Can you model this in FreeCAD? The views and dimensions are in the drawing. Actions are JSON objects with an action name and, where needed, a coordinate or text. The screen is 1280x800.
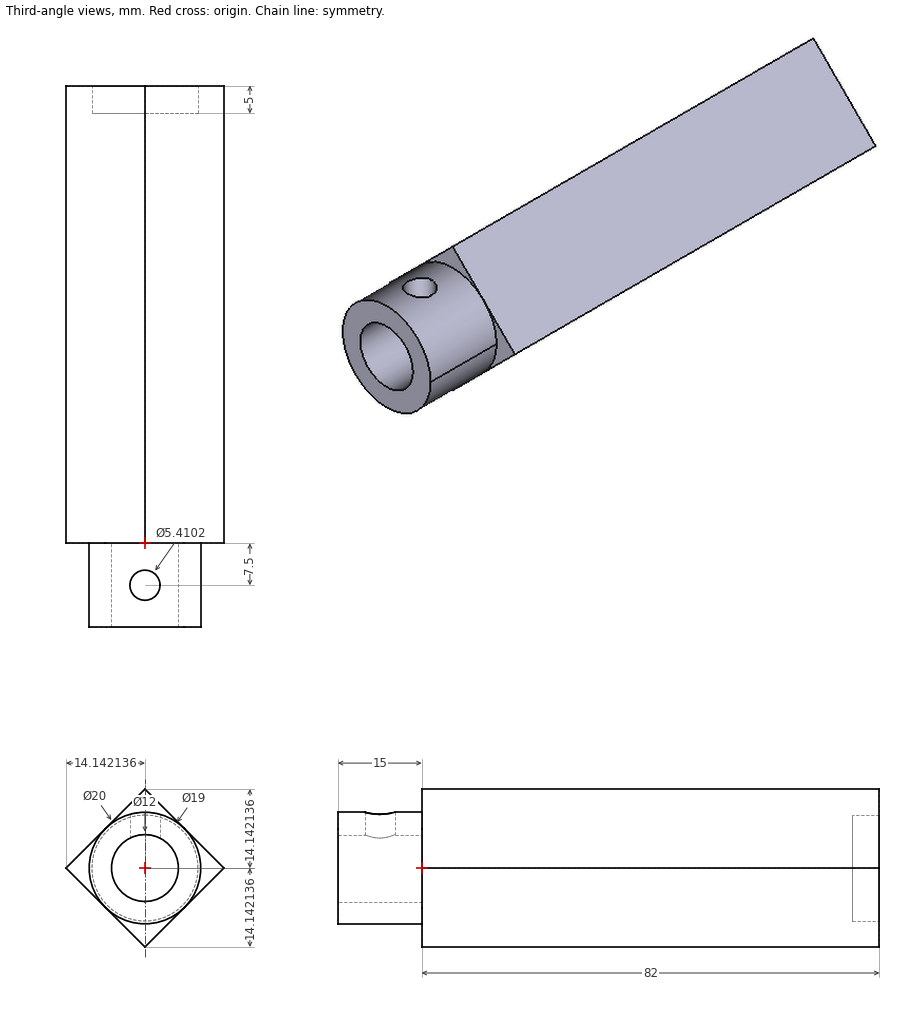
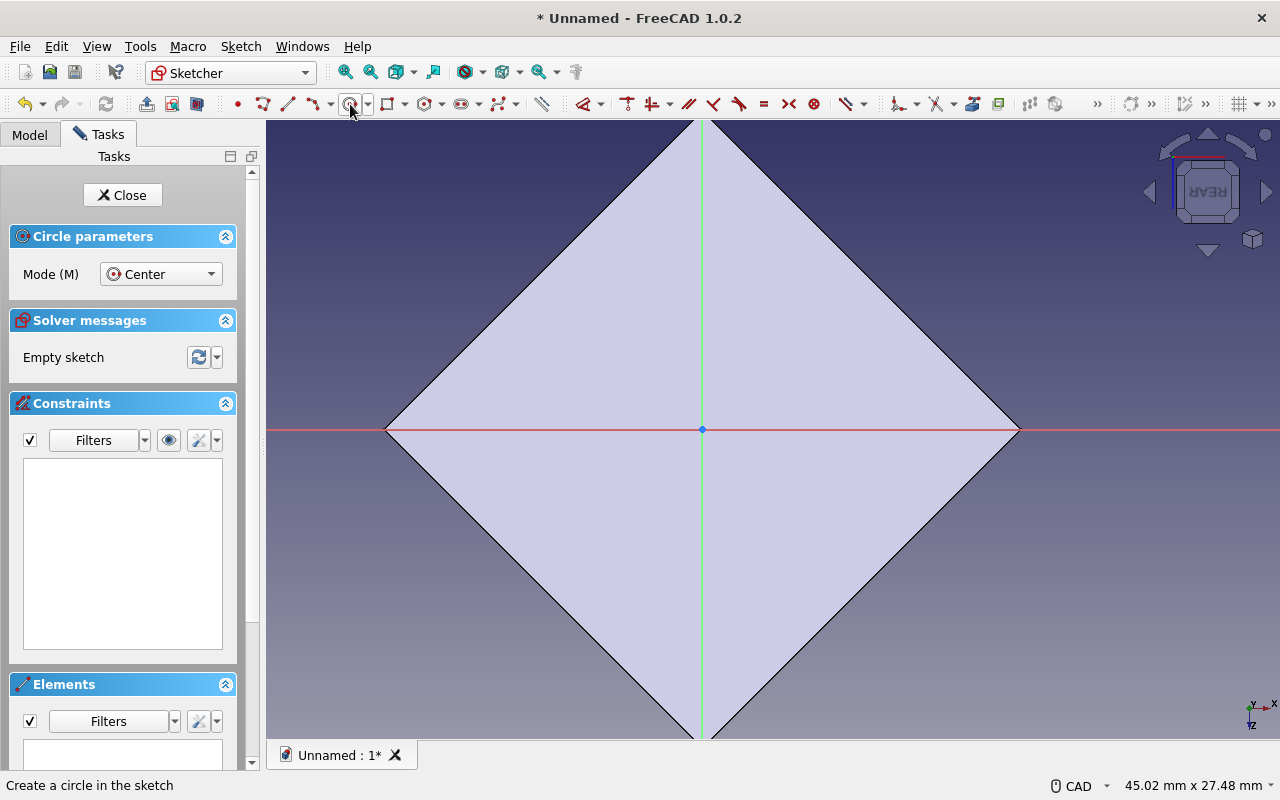
{"action": "left_click", "coordinate": [702, 429]}
{"action": "mouse_move", "coordinate": [853, 278]}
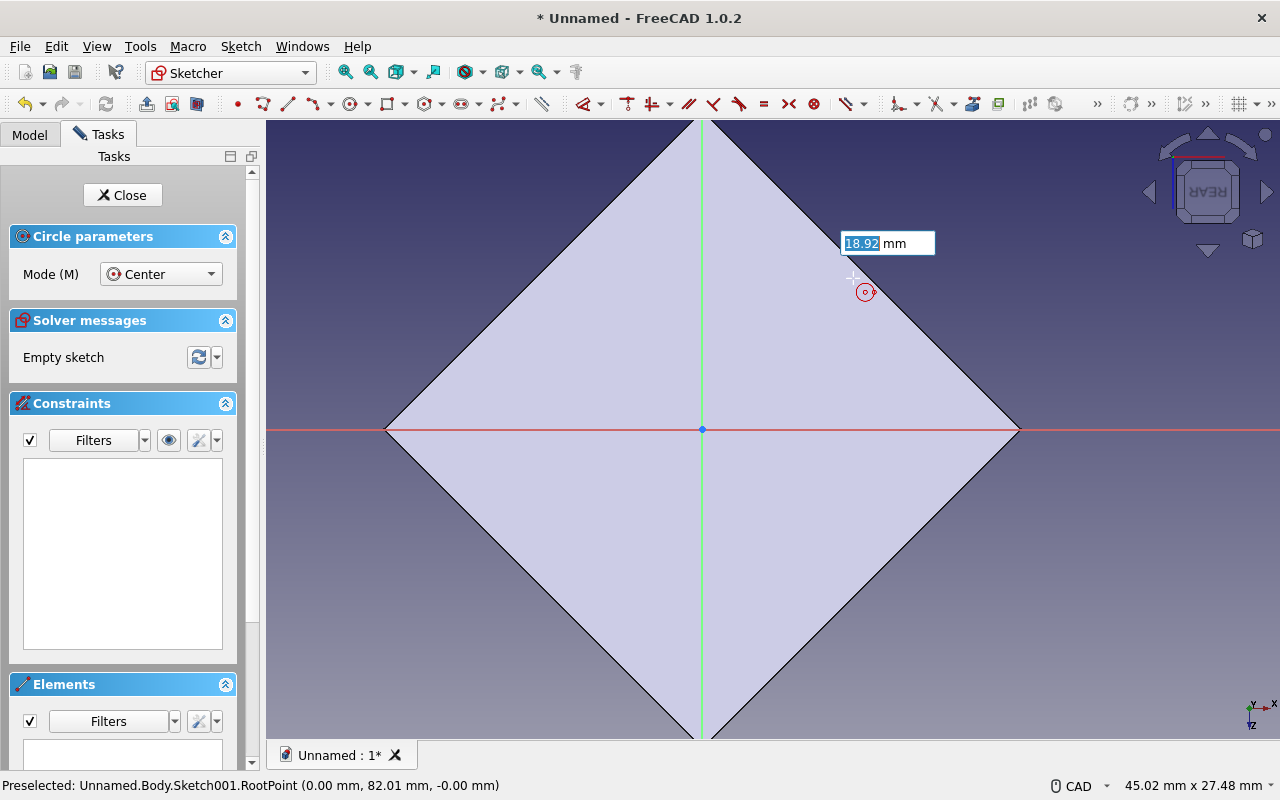
{"action": "type", "text": "19"}
{"action": "key", "text": "Return"}
{"action": "key", "text": "Escape"}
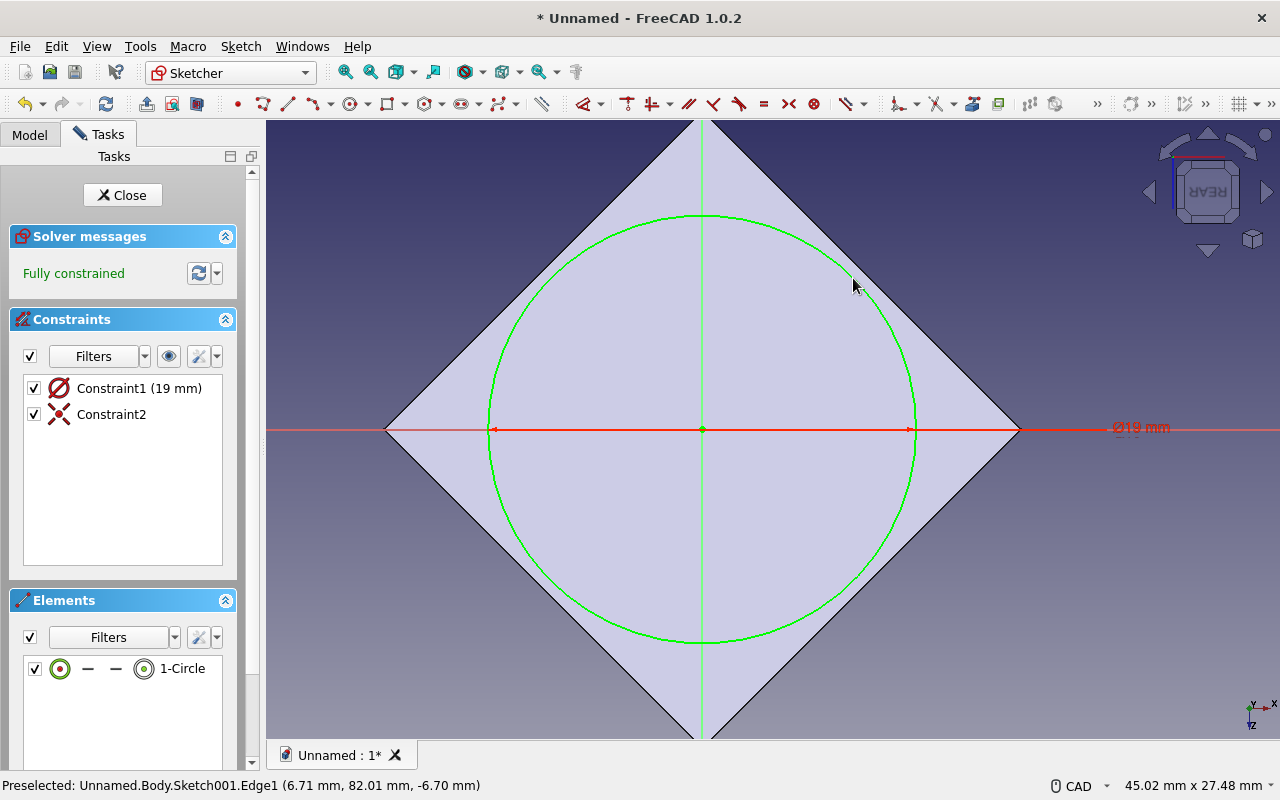
{"action": "left_click", "coordinate": [123, 195]}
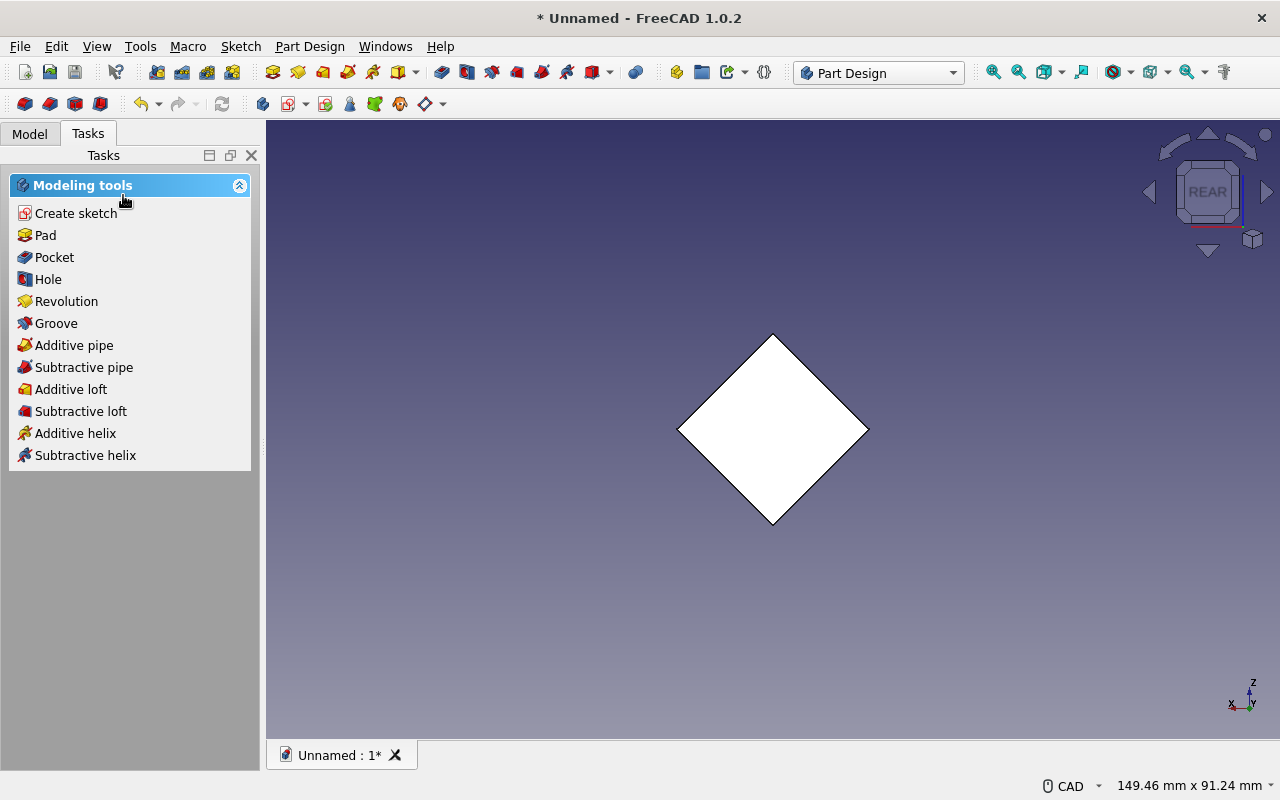
{"action": "left_click", "coordinate": [442, 72]}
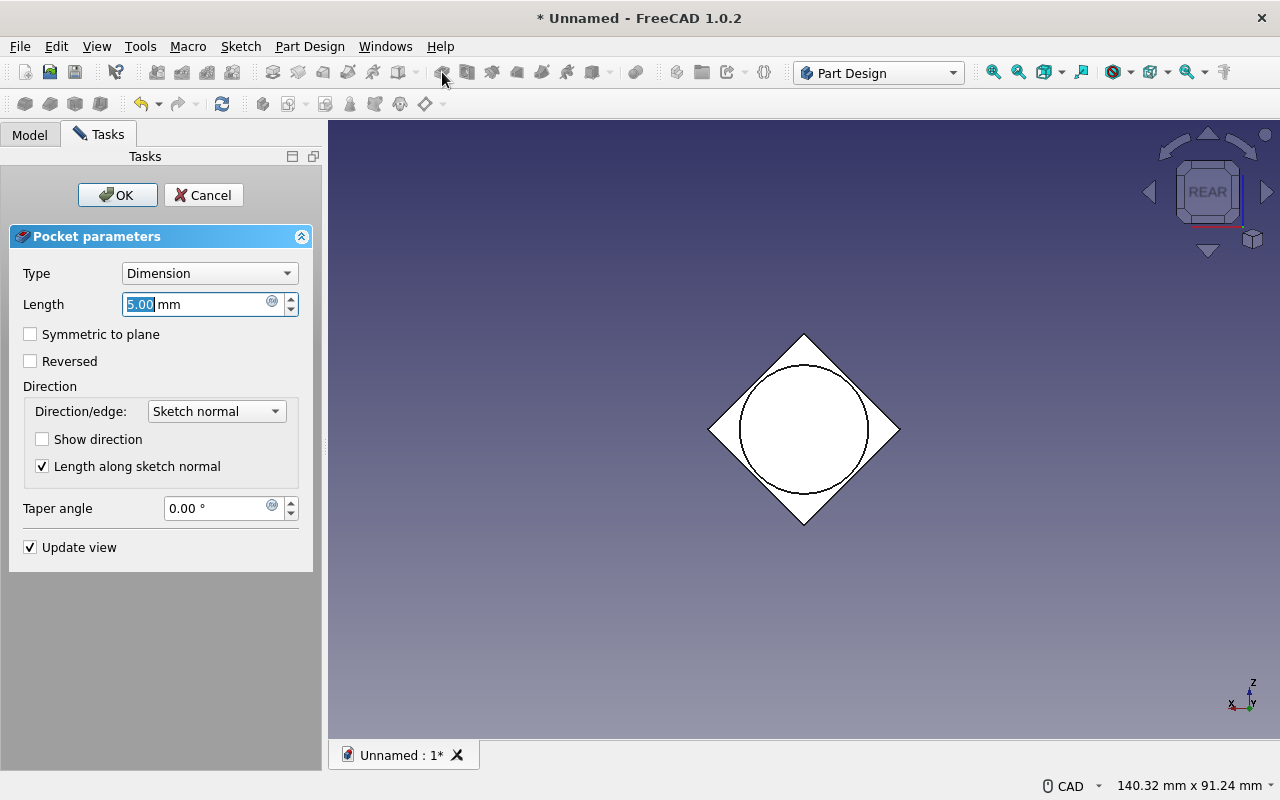
{"action": "type", "text": "5"}
{"action": "key", "text": "Tab"}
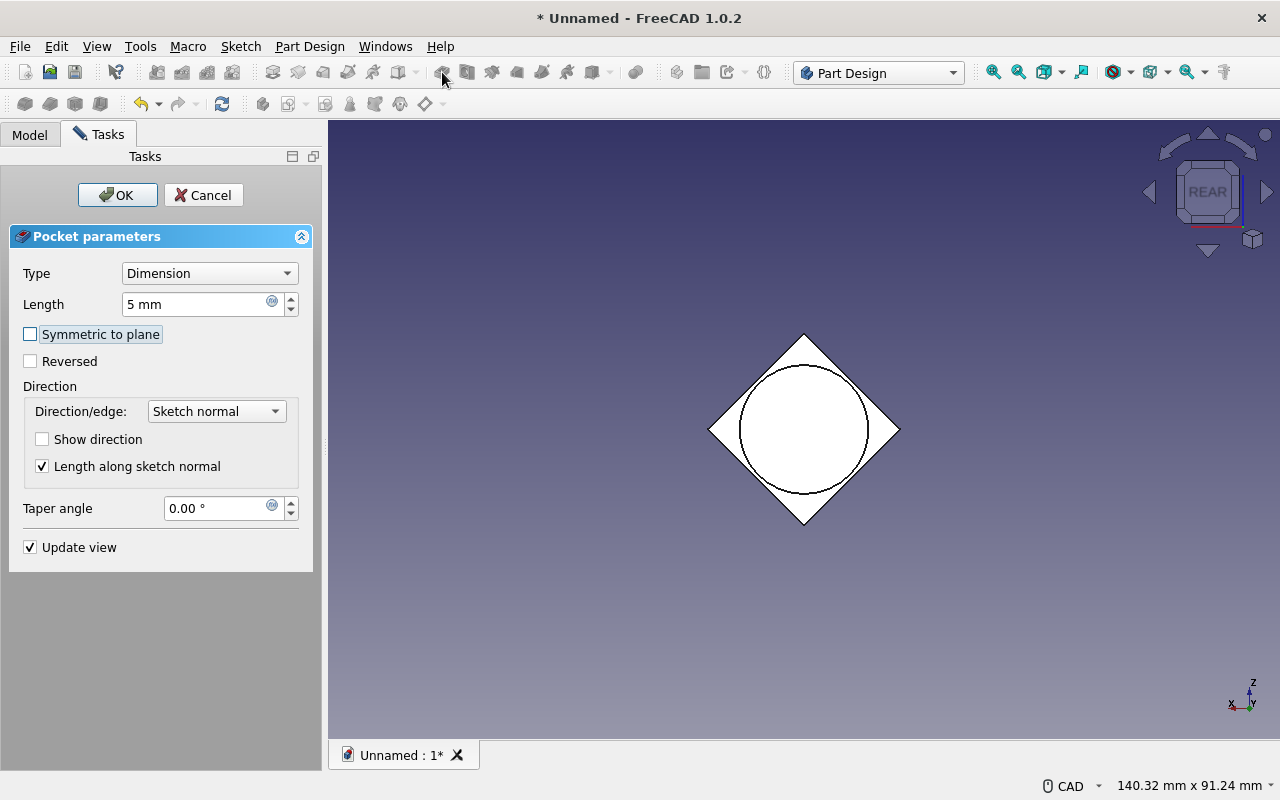
{"action": "left_click", "coordinate": [118, 195]}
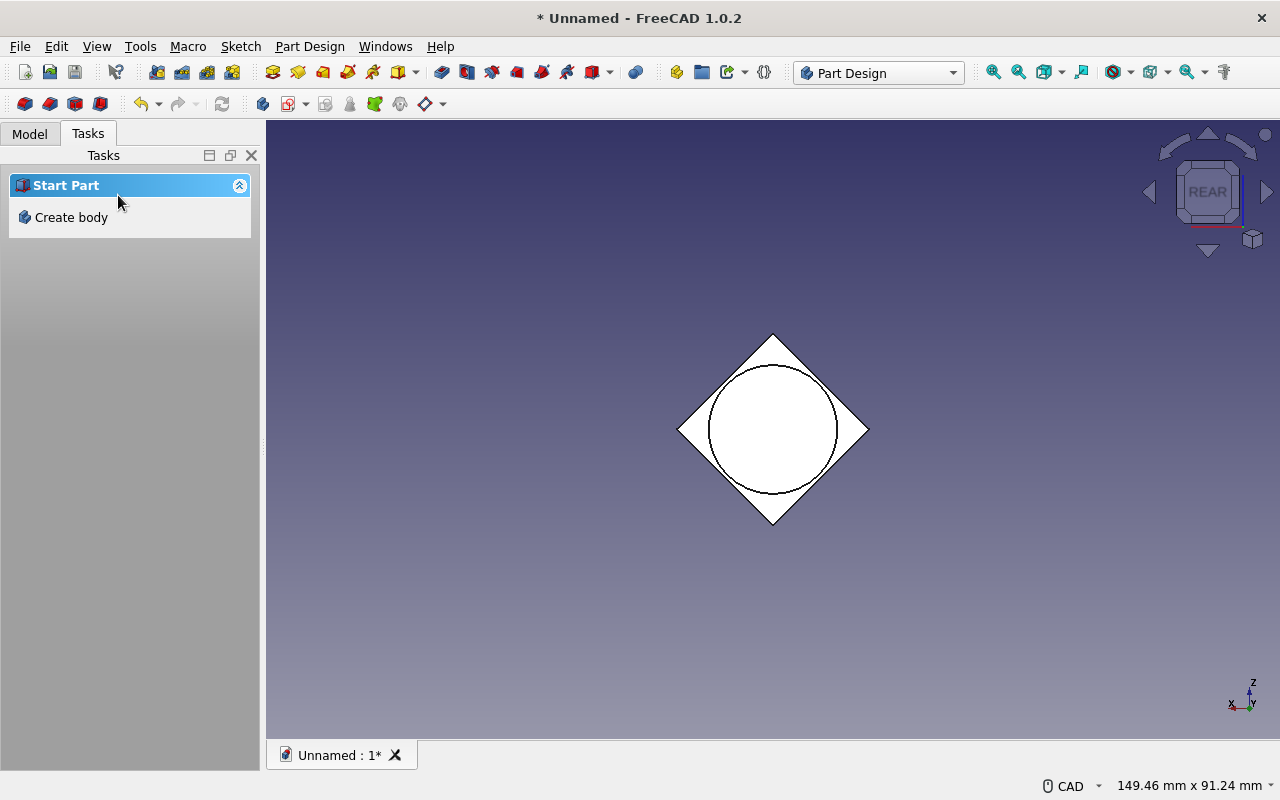
{"action": "key", "text": "v f"}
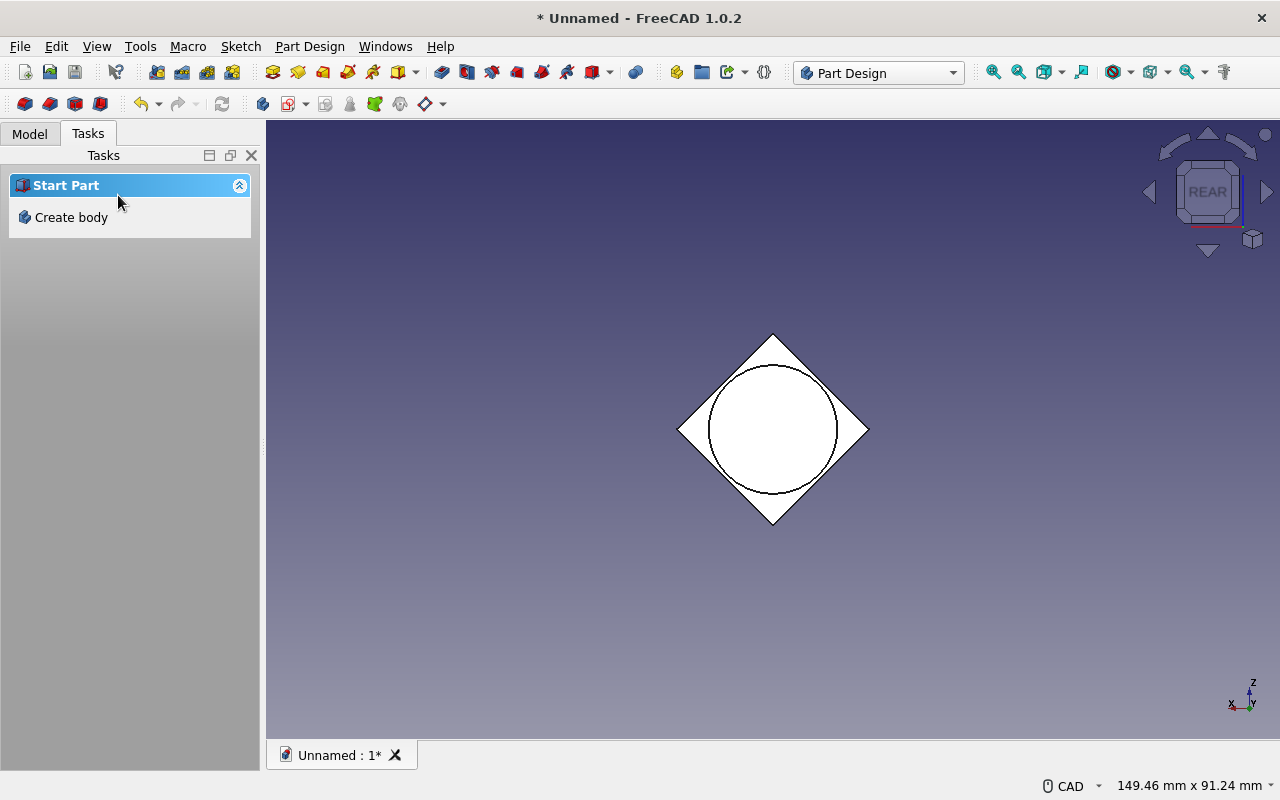
{"action": "key", "text": "0"}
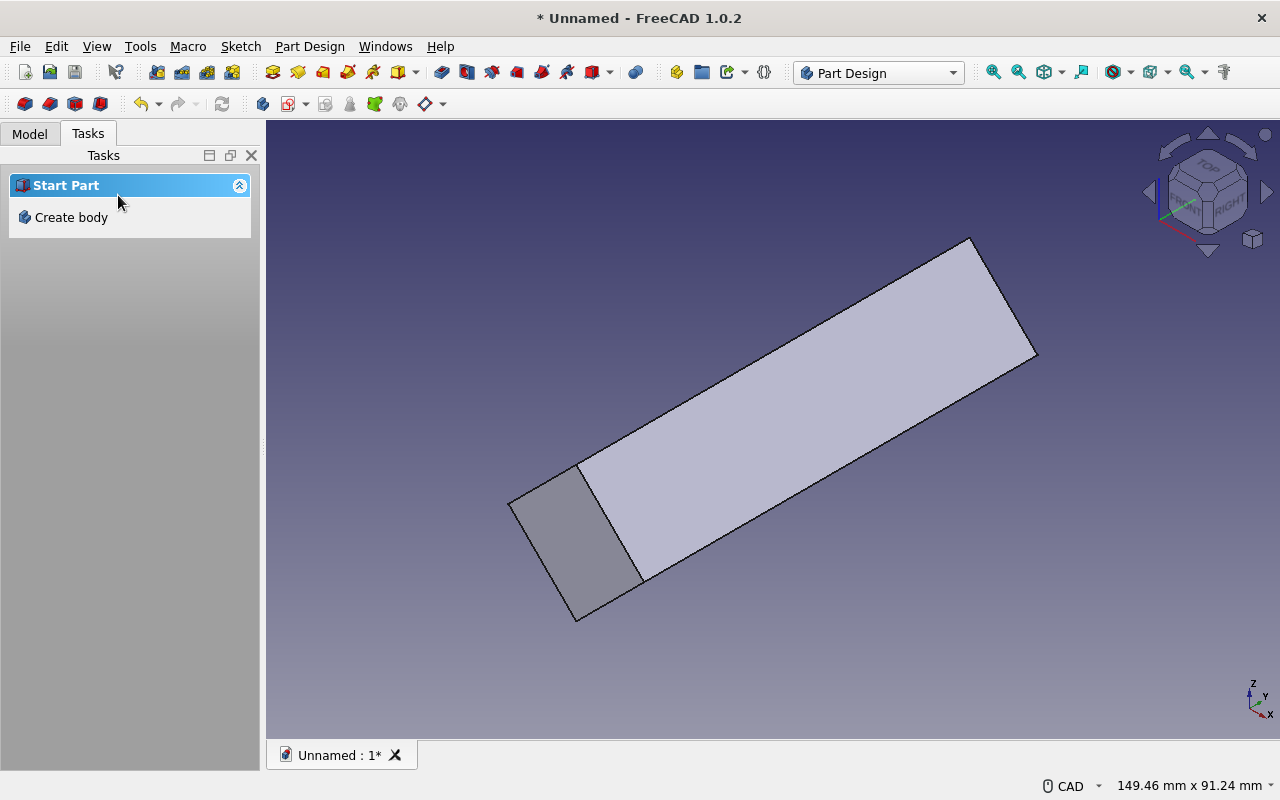
{"action": "left_click", "coordinate": [576, 542]}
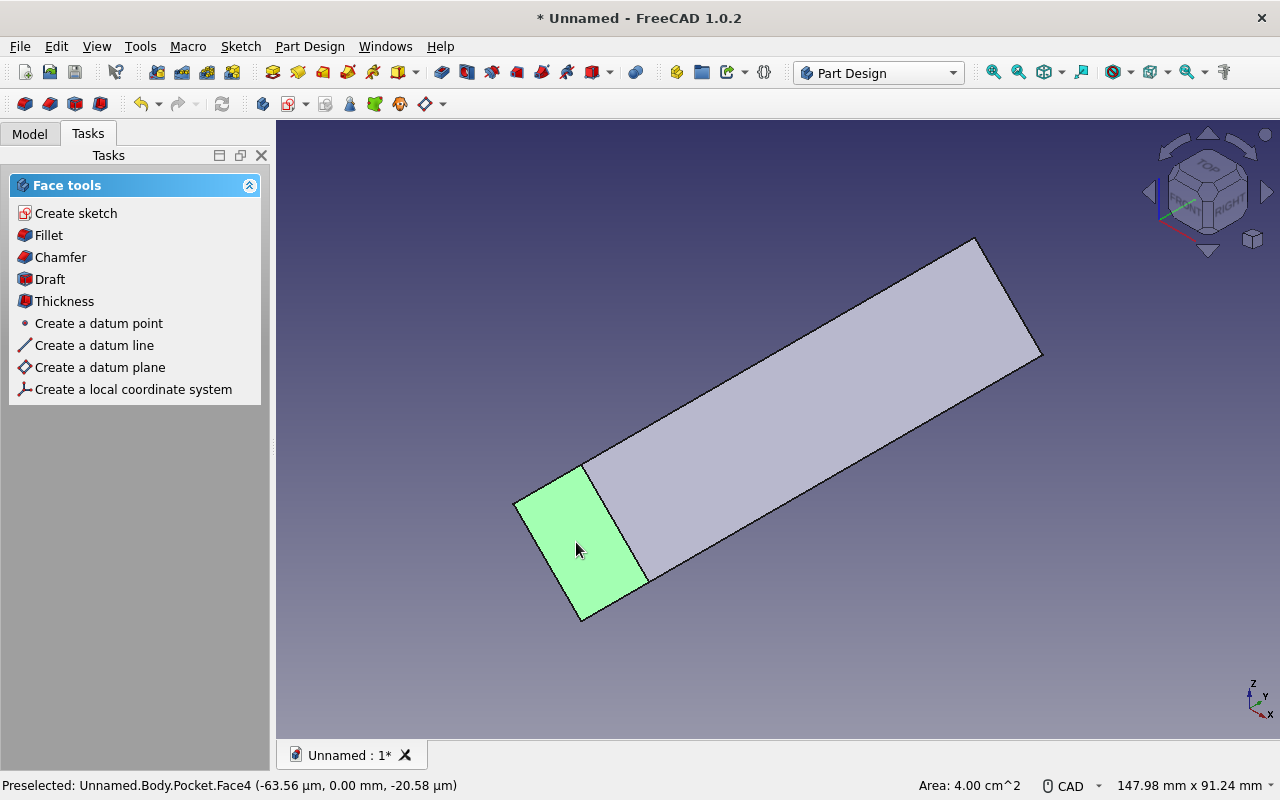
{"action": "left_click", "coordinate": [288, 104]}